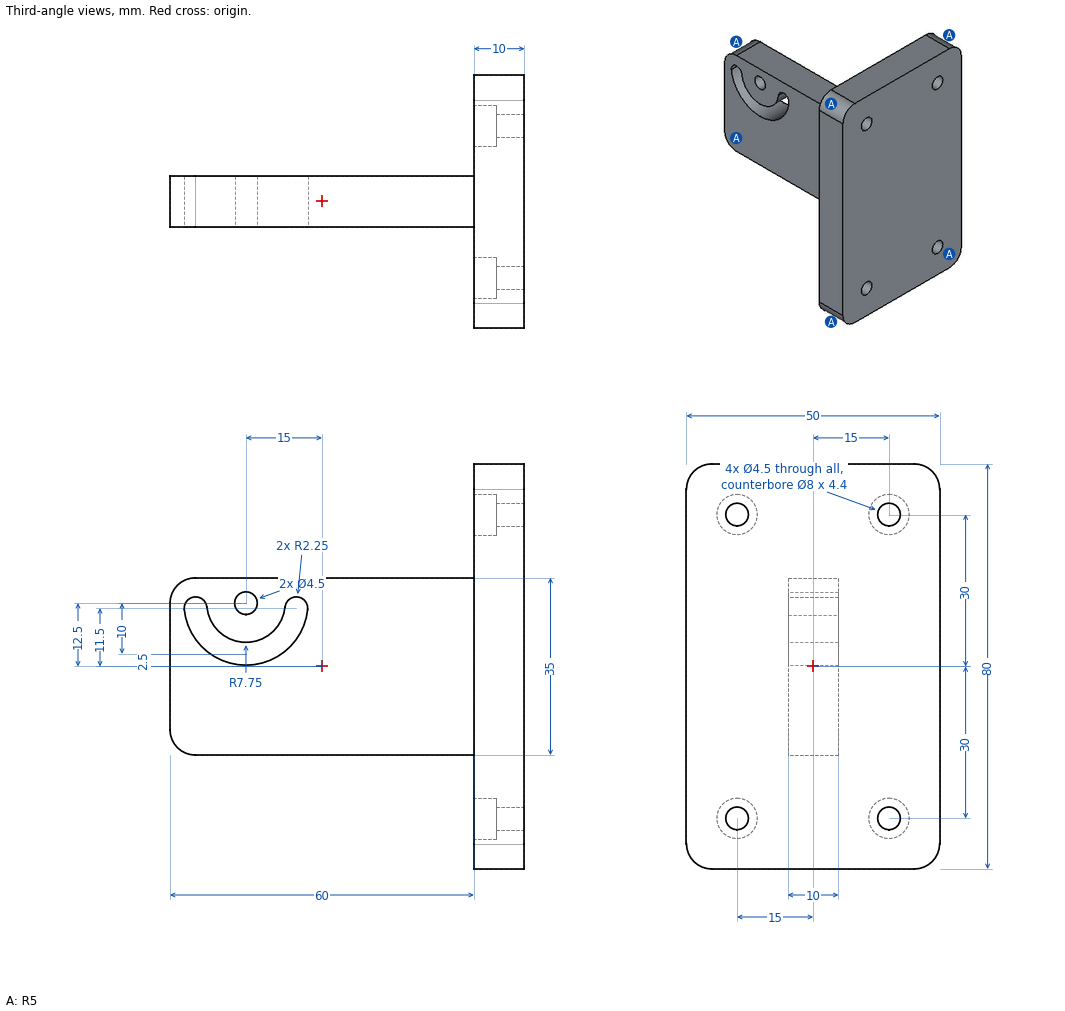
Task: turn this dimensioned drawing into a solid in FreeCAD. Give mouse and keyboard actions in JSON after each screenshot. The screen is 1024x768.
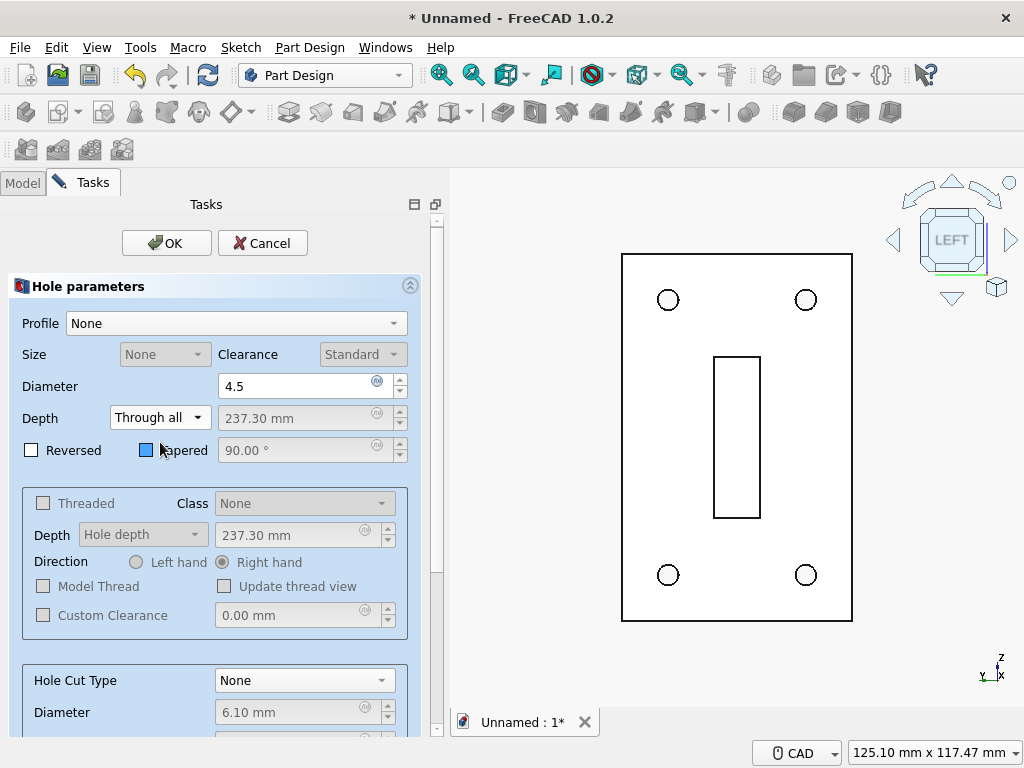
{"action": "left_click", "coordinate": [306, 680]}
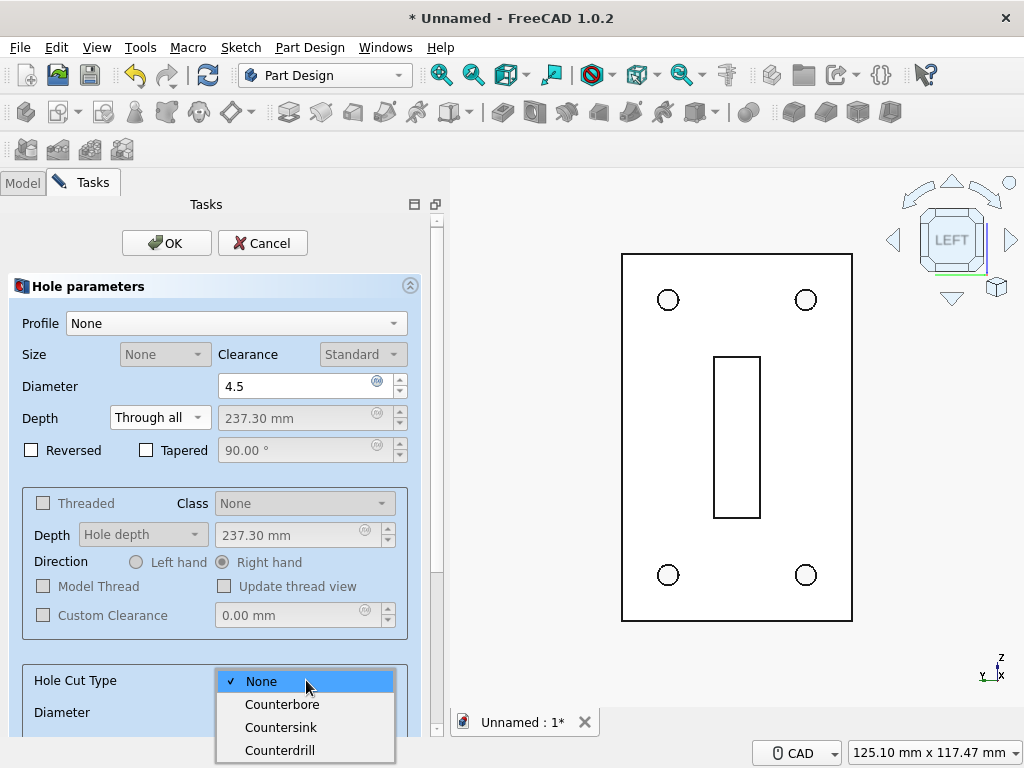
{"action": "left_click", "coordinate": [304, 704]}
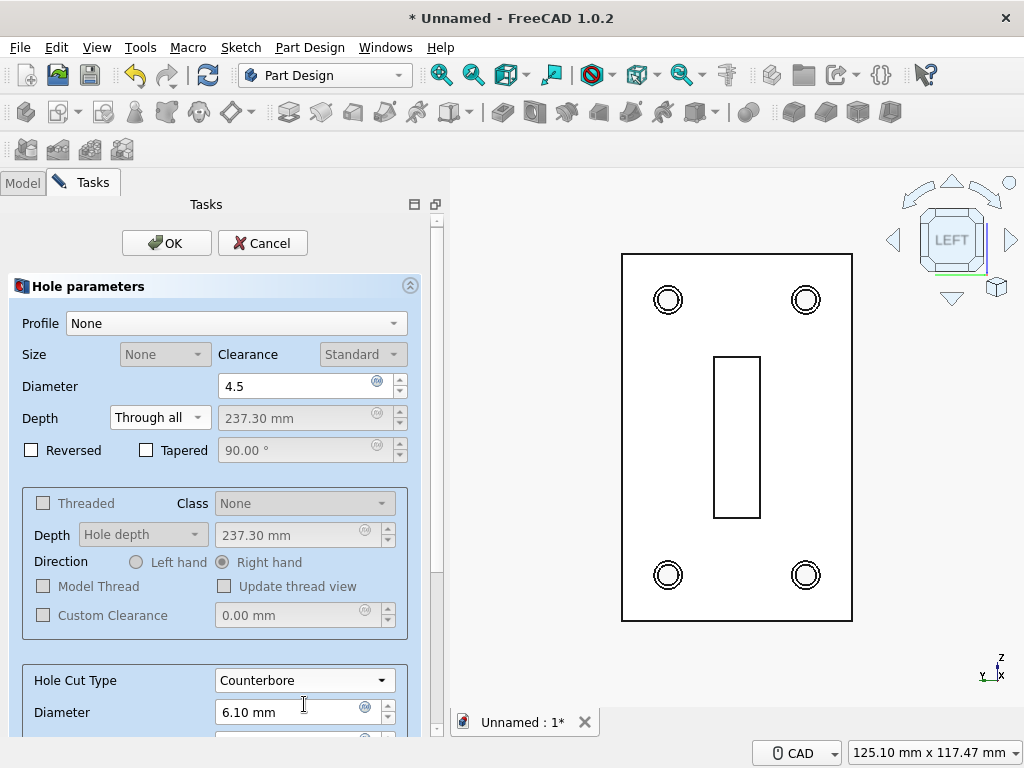
{"action": "triple_click", "coordinate": [298, 712]}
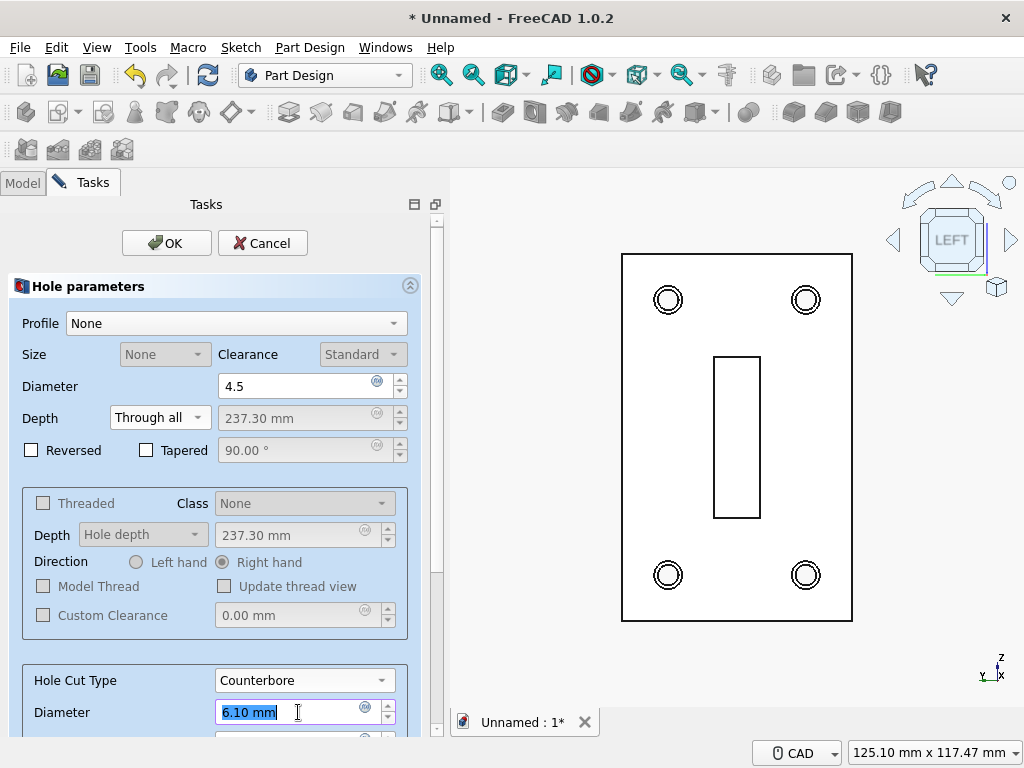
{"action": "type", "text": "8"}
{"action": "key", "text": "Tab"}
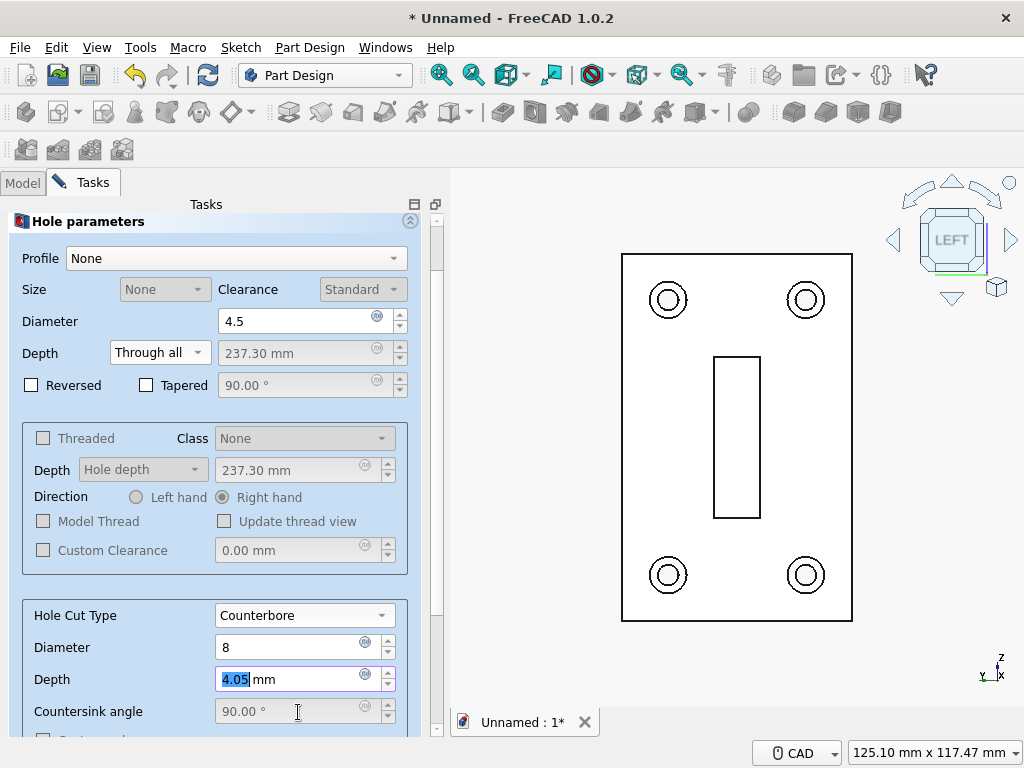
{"action": "type", "text": "4.4"}
{"action": "key", "text": "Tab"}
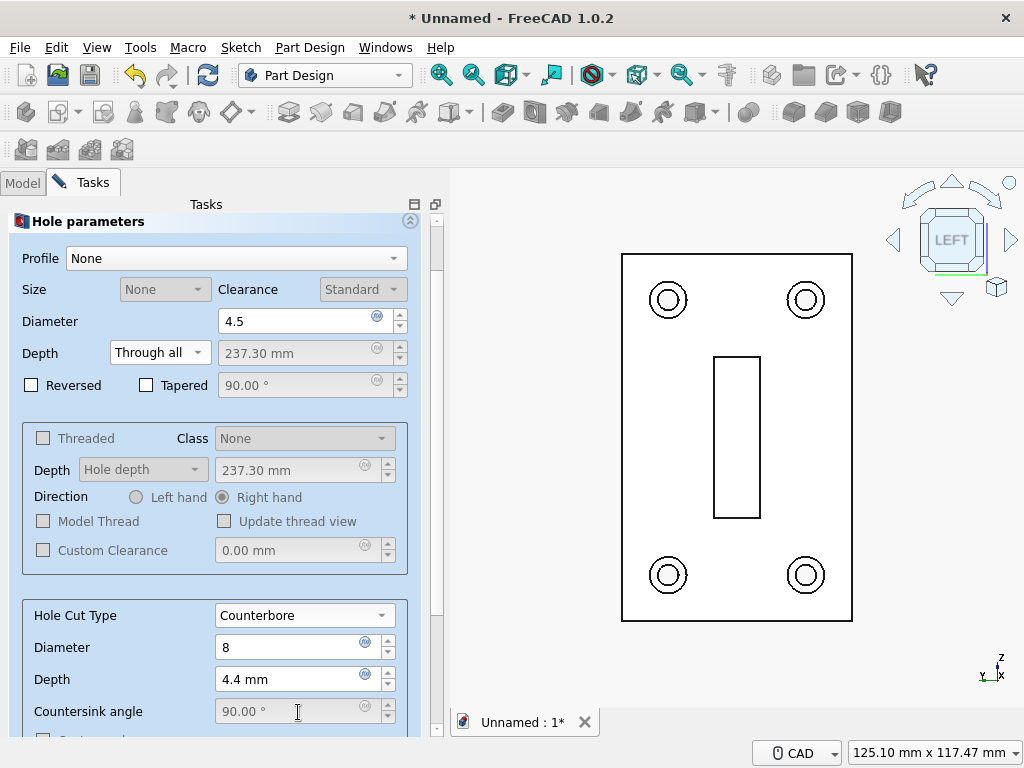
{"action": "scroll", "coordinate": [437, 475], "scroll_direction": "up", "scroll_amount": 2}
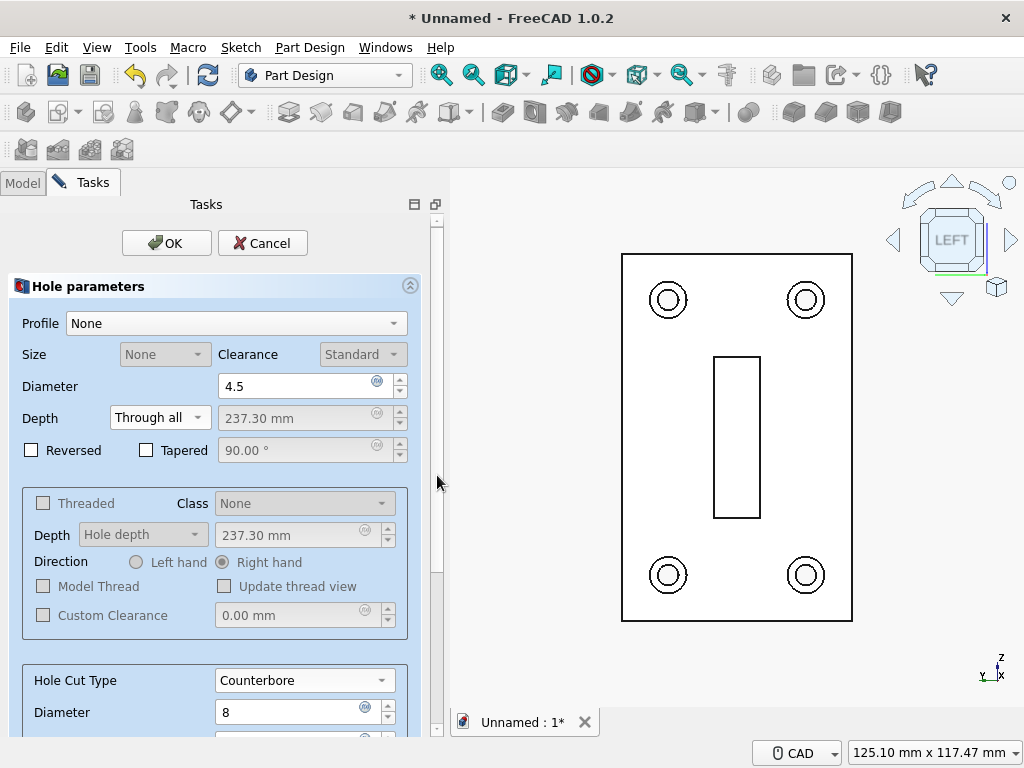
{"action": "left_click", "coordinate": [167, 243]}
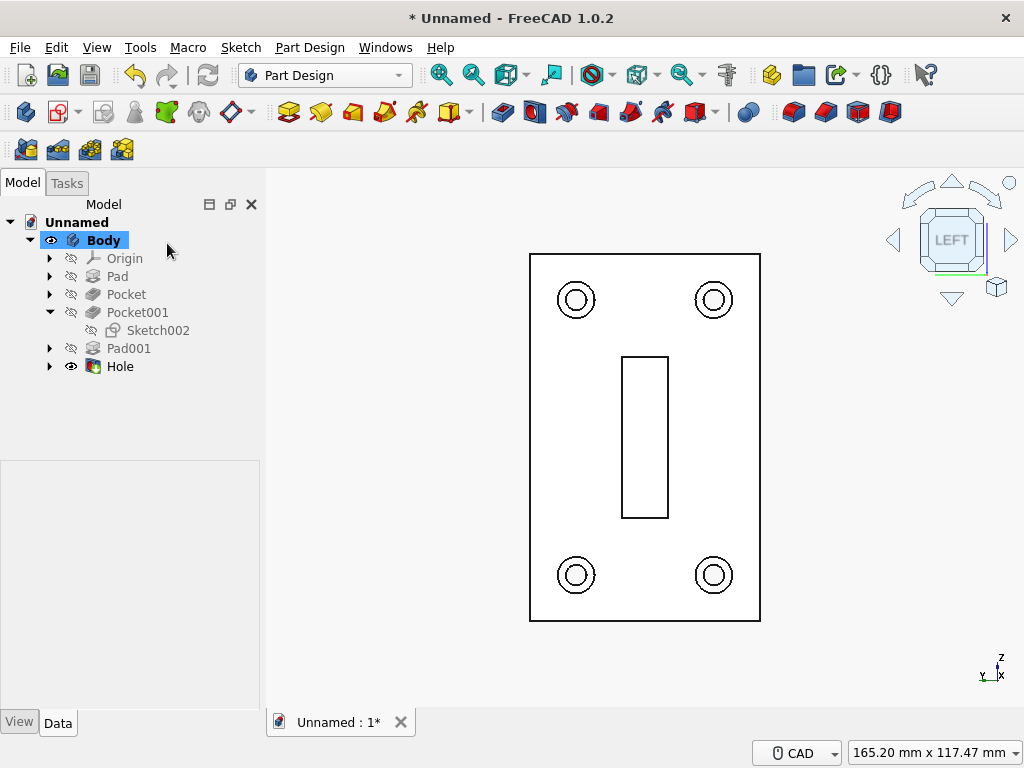
{"action": "left_click", "coordinate": [645, 356]}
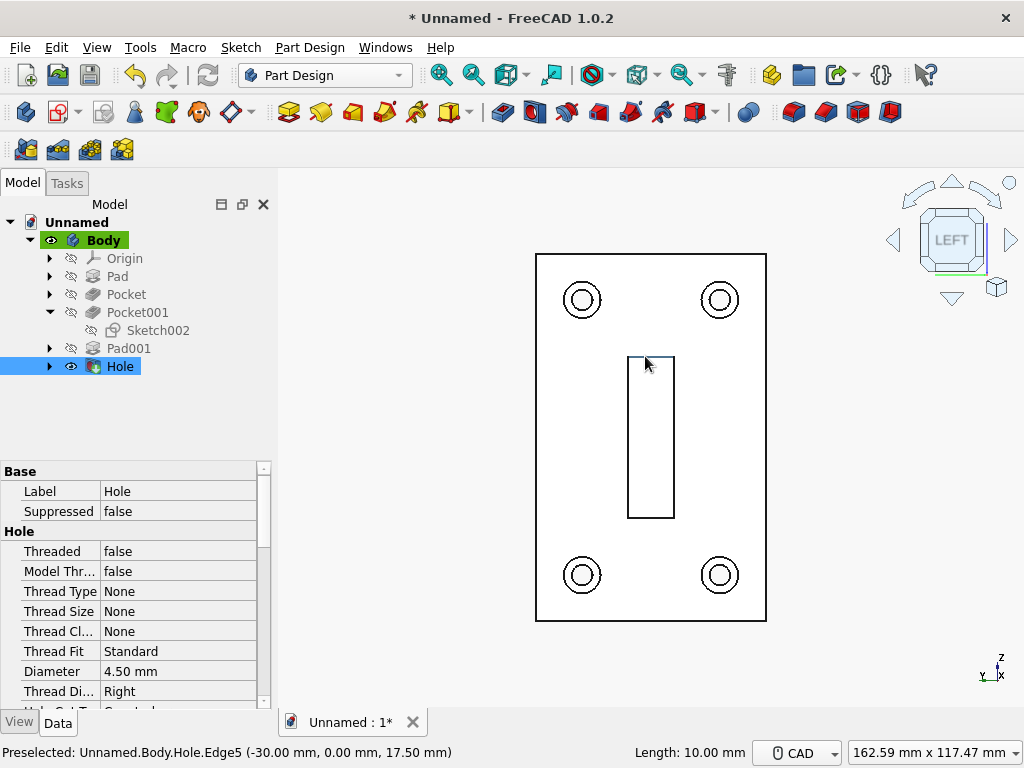
{"action": "left_click", "coordinate": [651, 517], "text": "ctrl"}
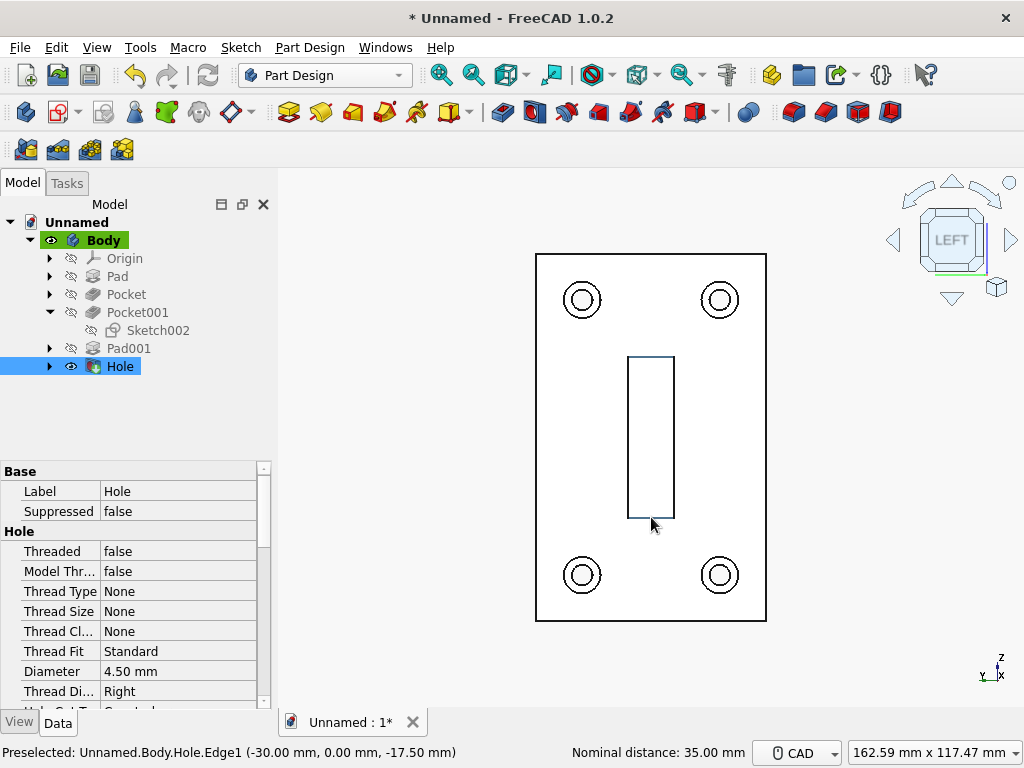
{"action": "key", "text": "0"}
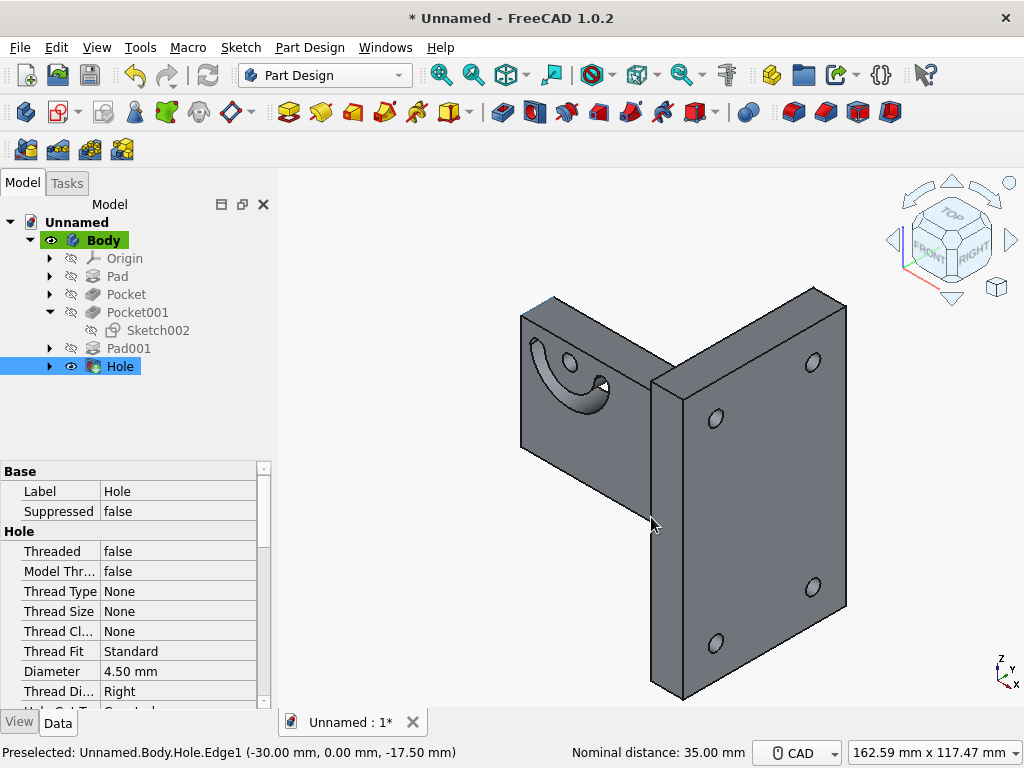
{"action": "left_click", "coordinate": [667, 390], "text": "ctrl"}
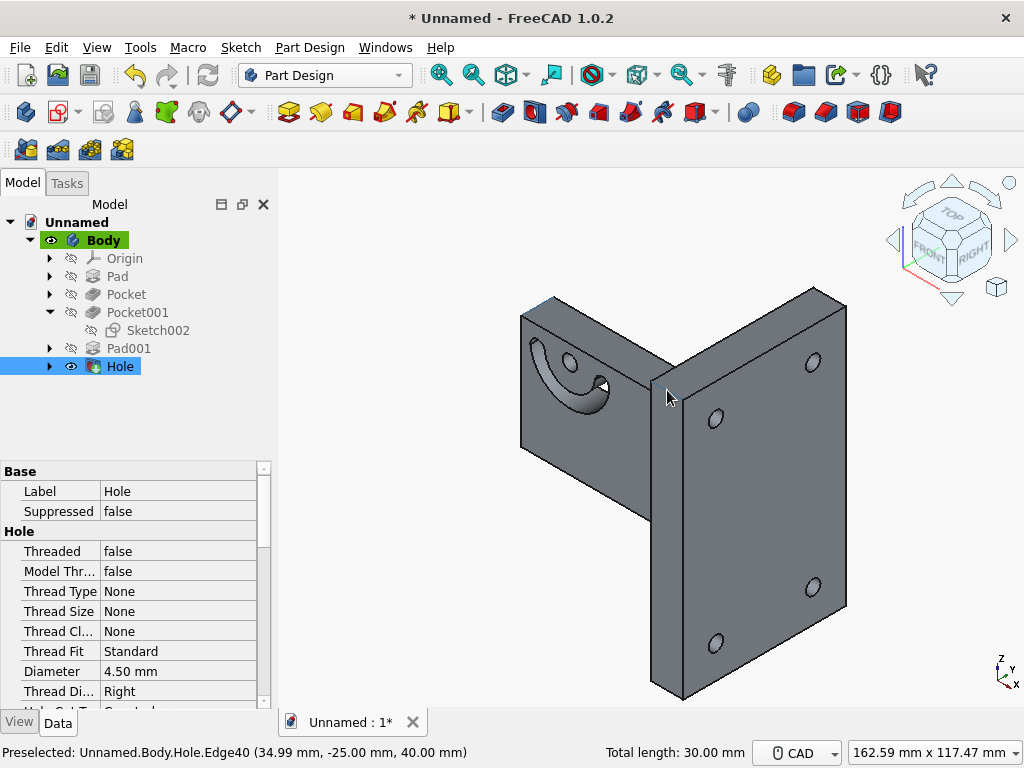
{"action": "key", "text": "2"}